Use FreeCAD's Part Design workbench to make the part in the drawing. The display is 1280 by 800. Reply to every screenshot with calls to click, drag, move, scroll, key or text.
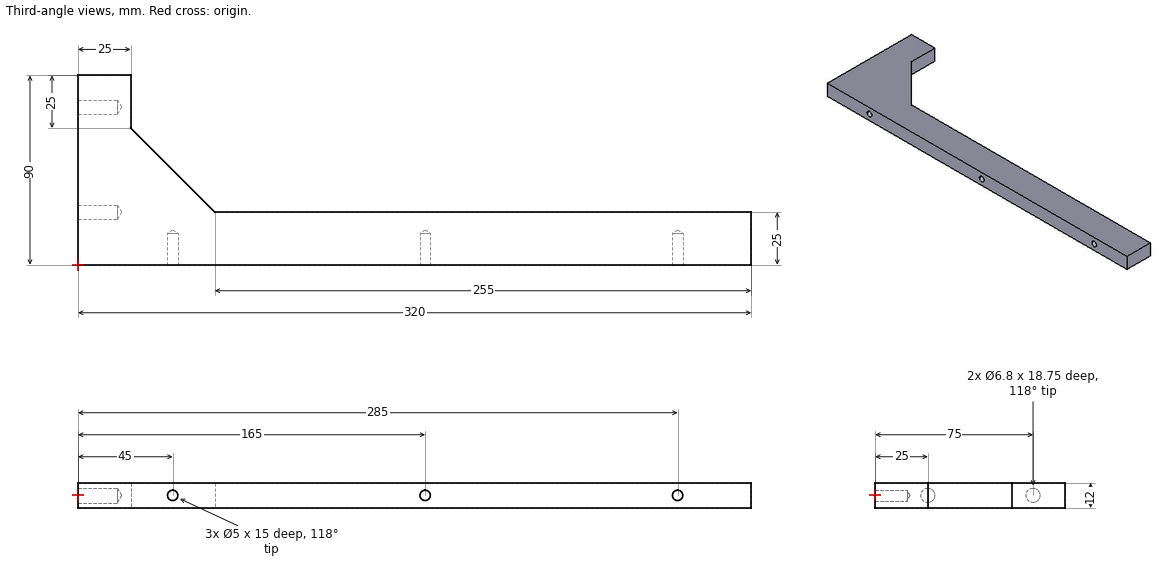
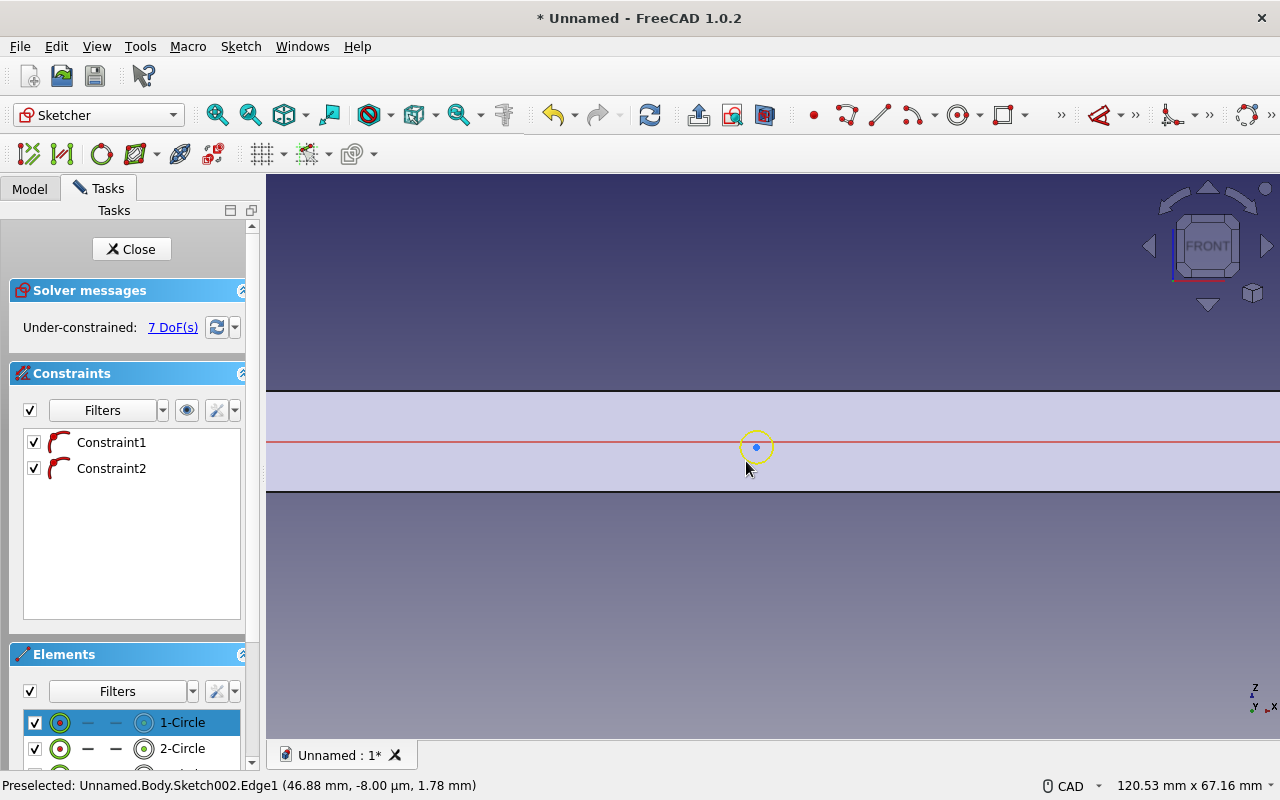
click(745, 459)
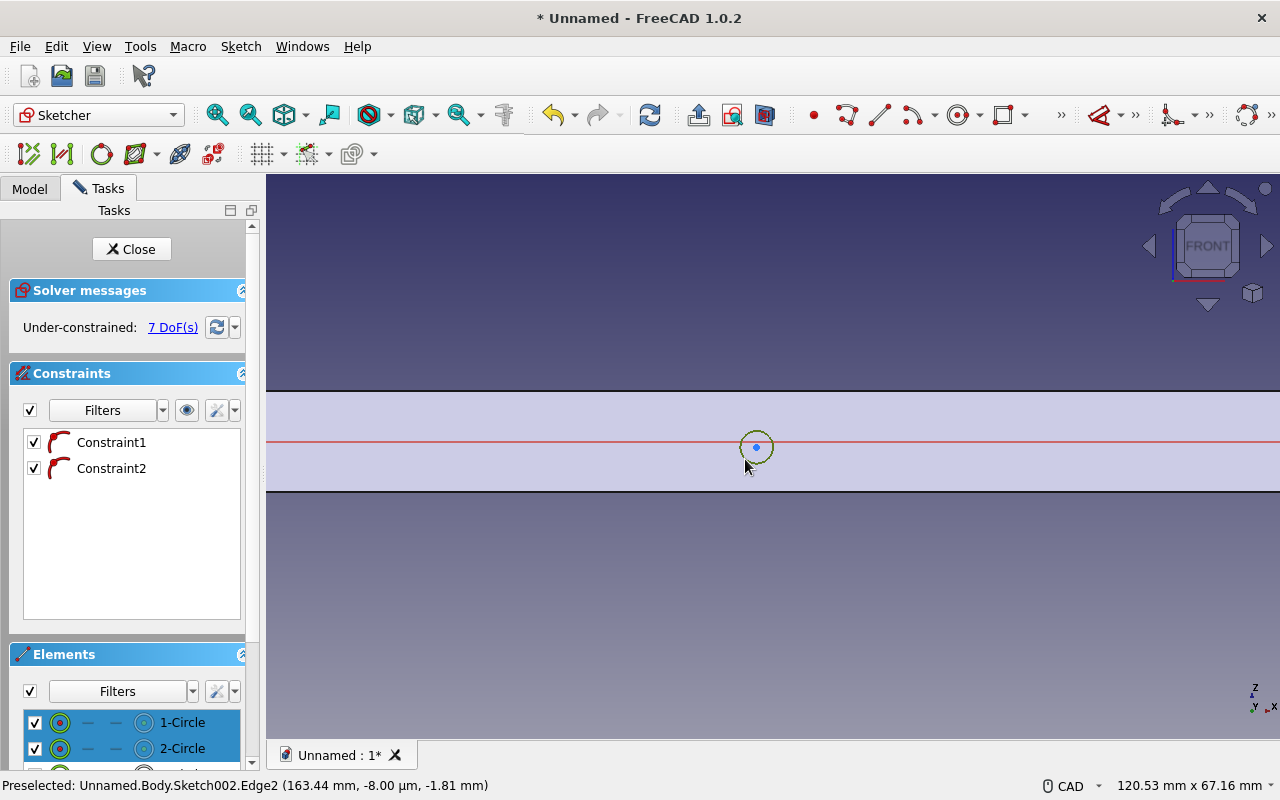
scroll(746, 461, down, 7)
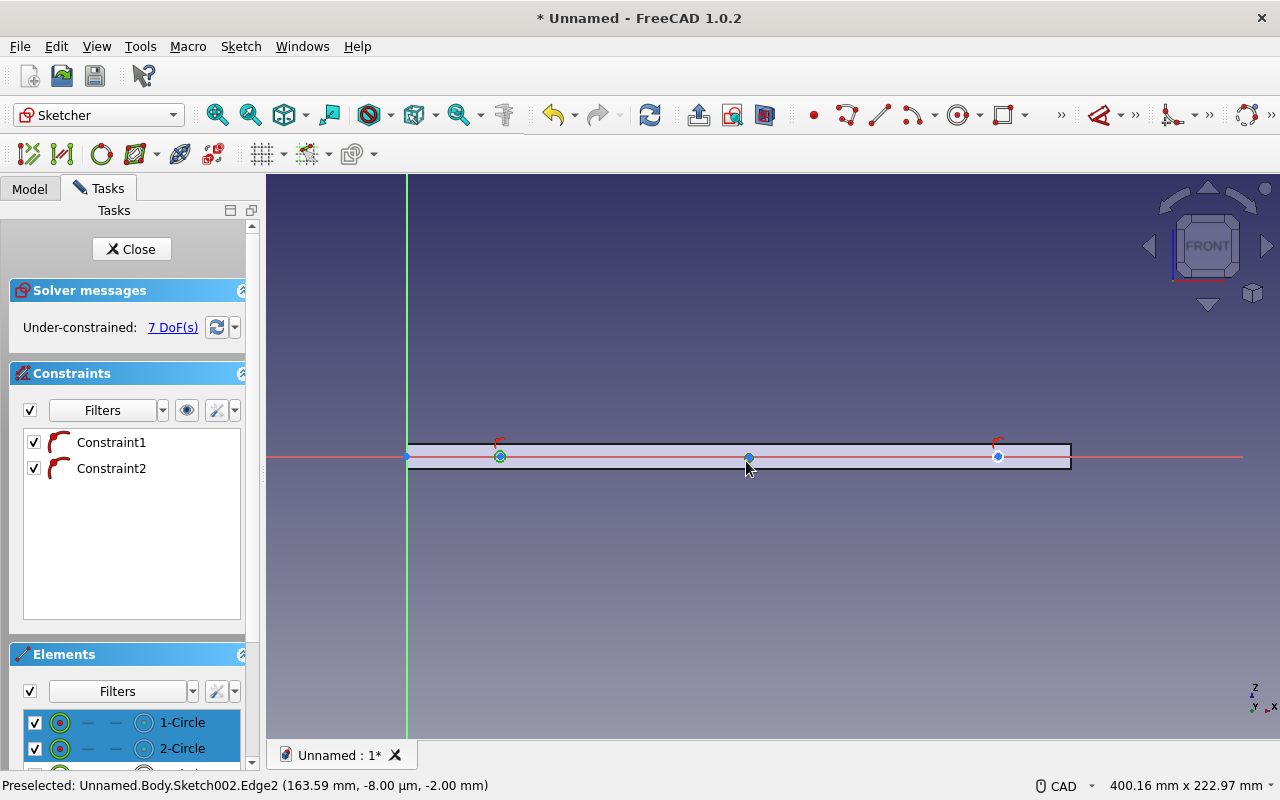
scroll(1002, 453, up, 7)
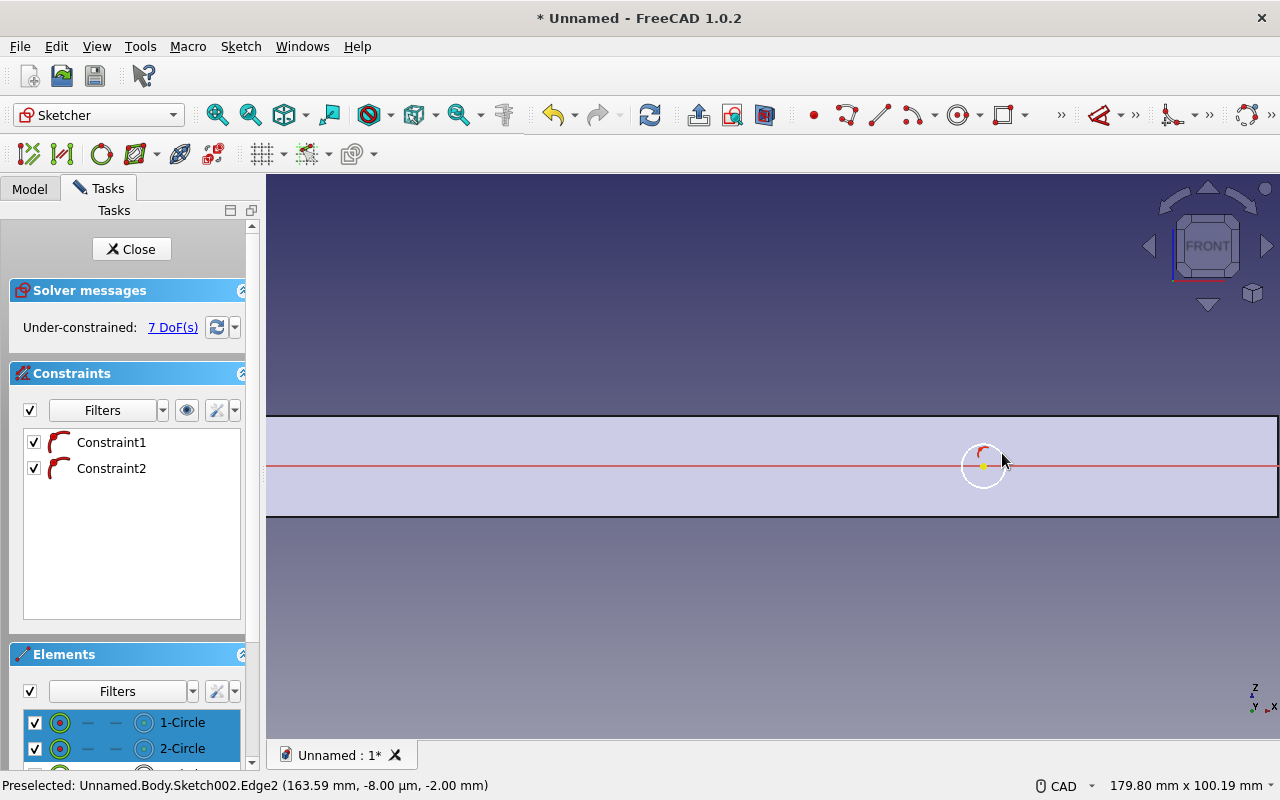
click(999, 451)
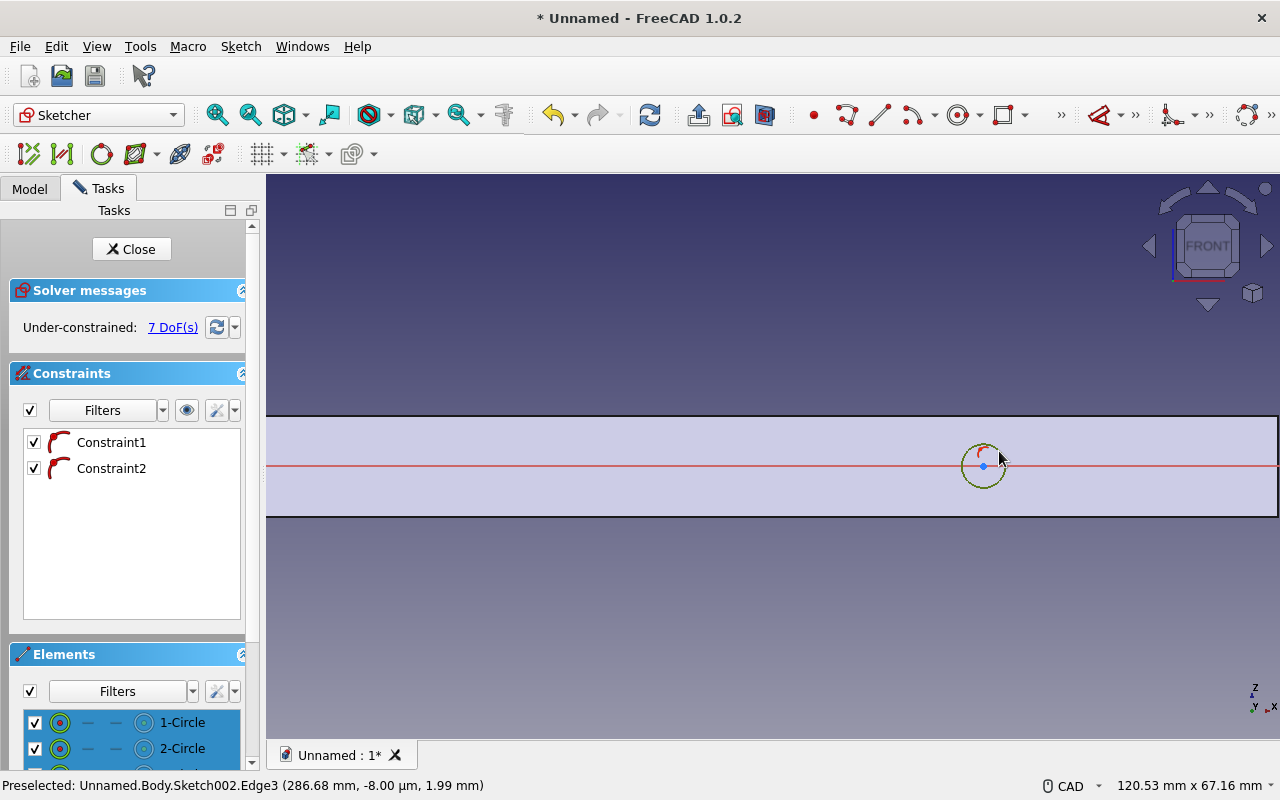
key(e)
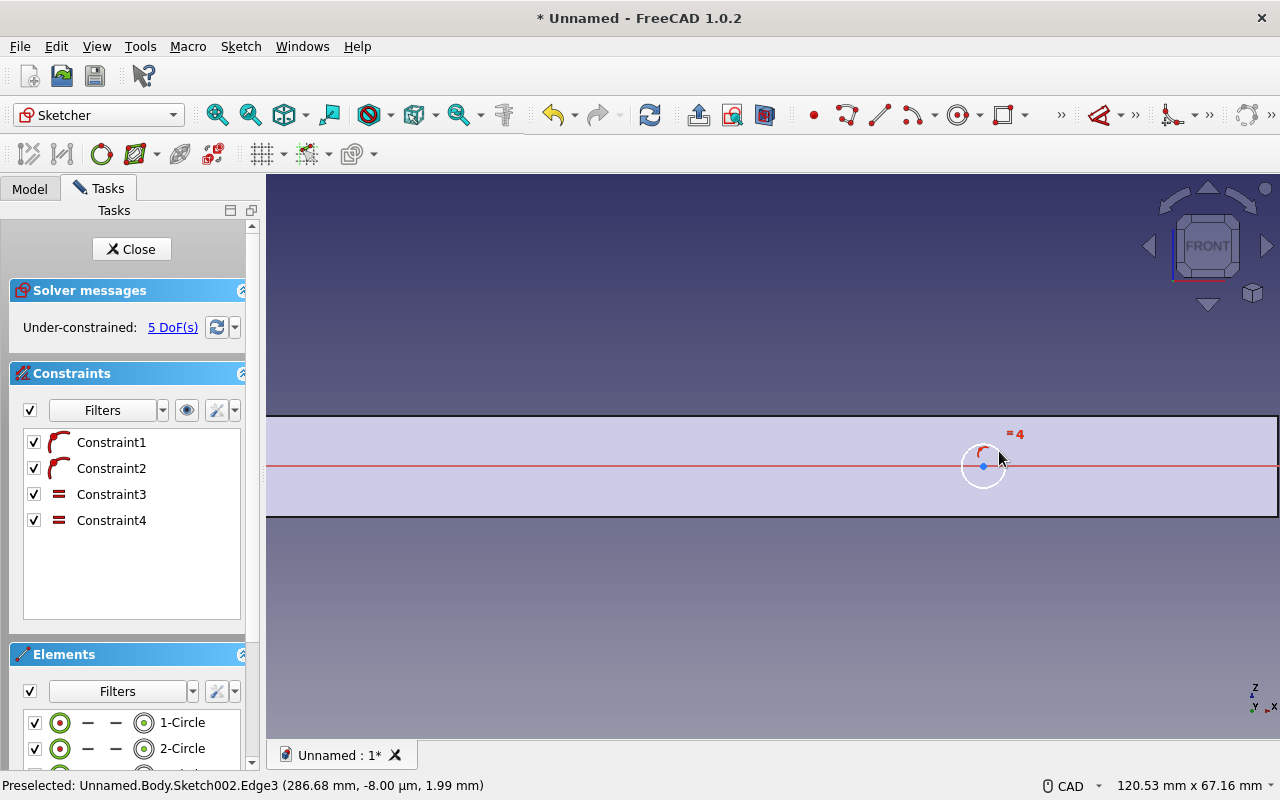
scroll(1002, 453, down, 7)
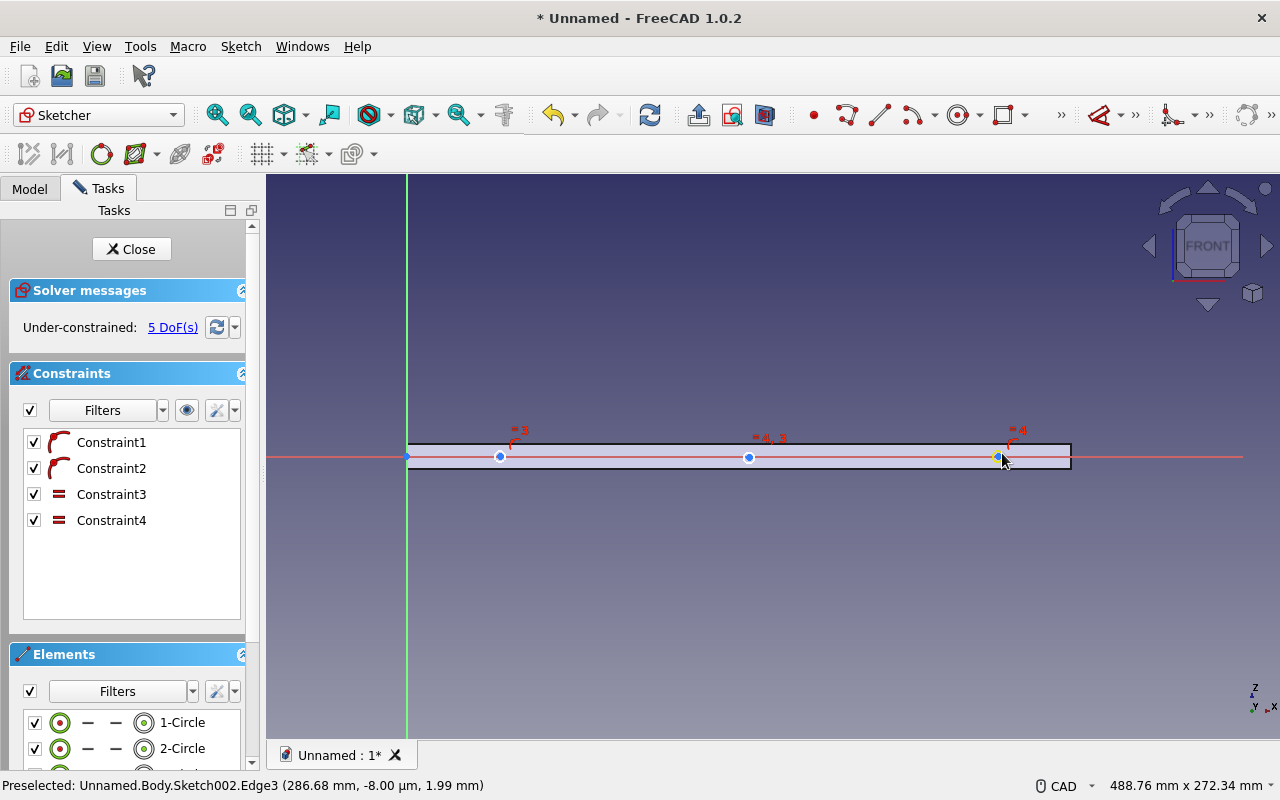
click(749, 458)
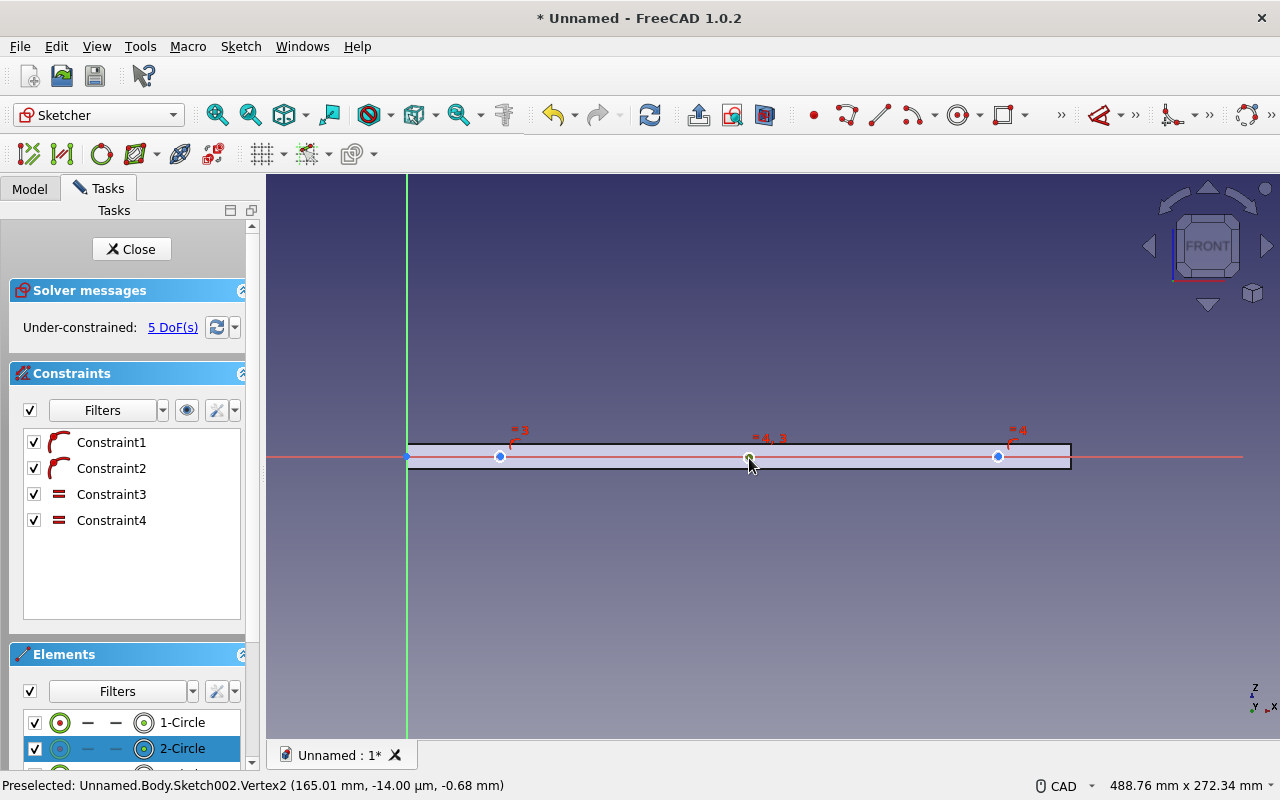
click(353, 457)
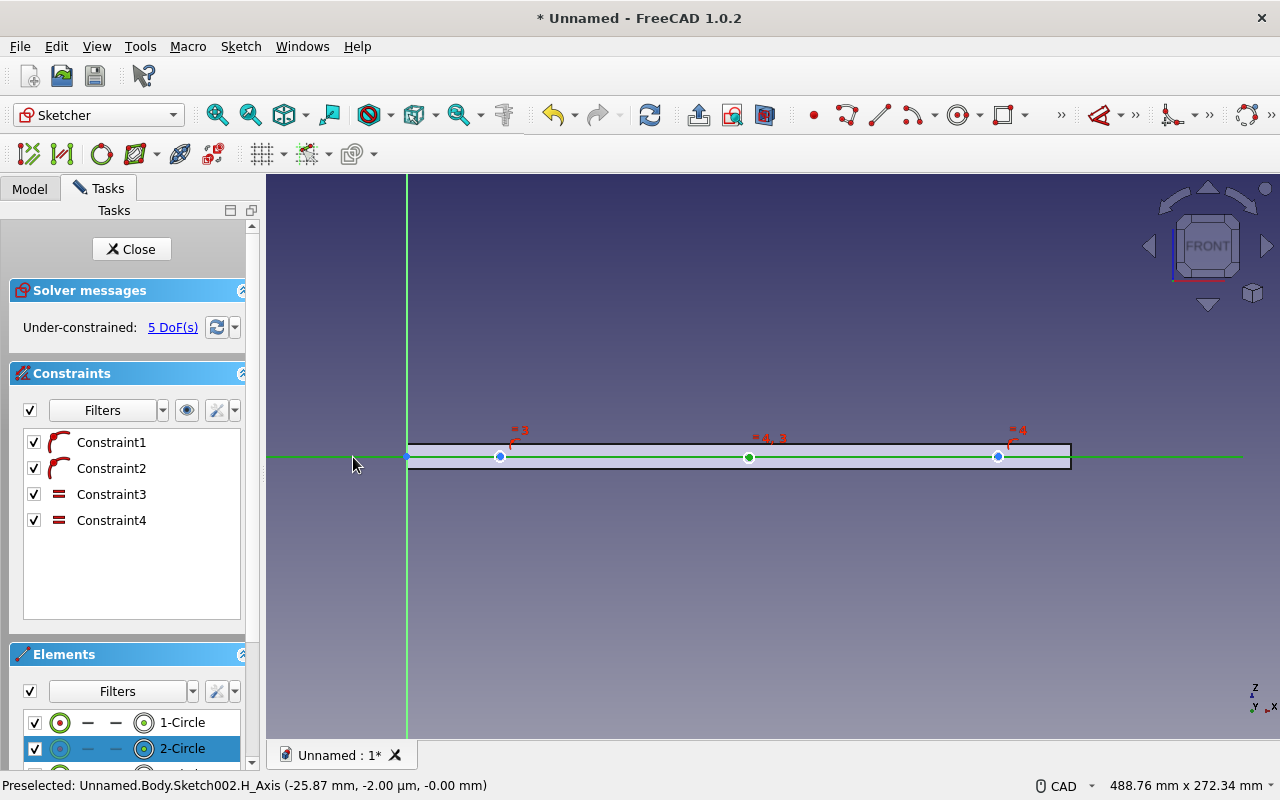
key(c)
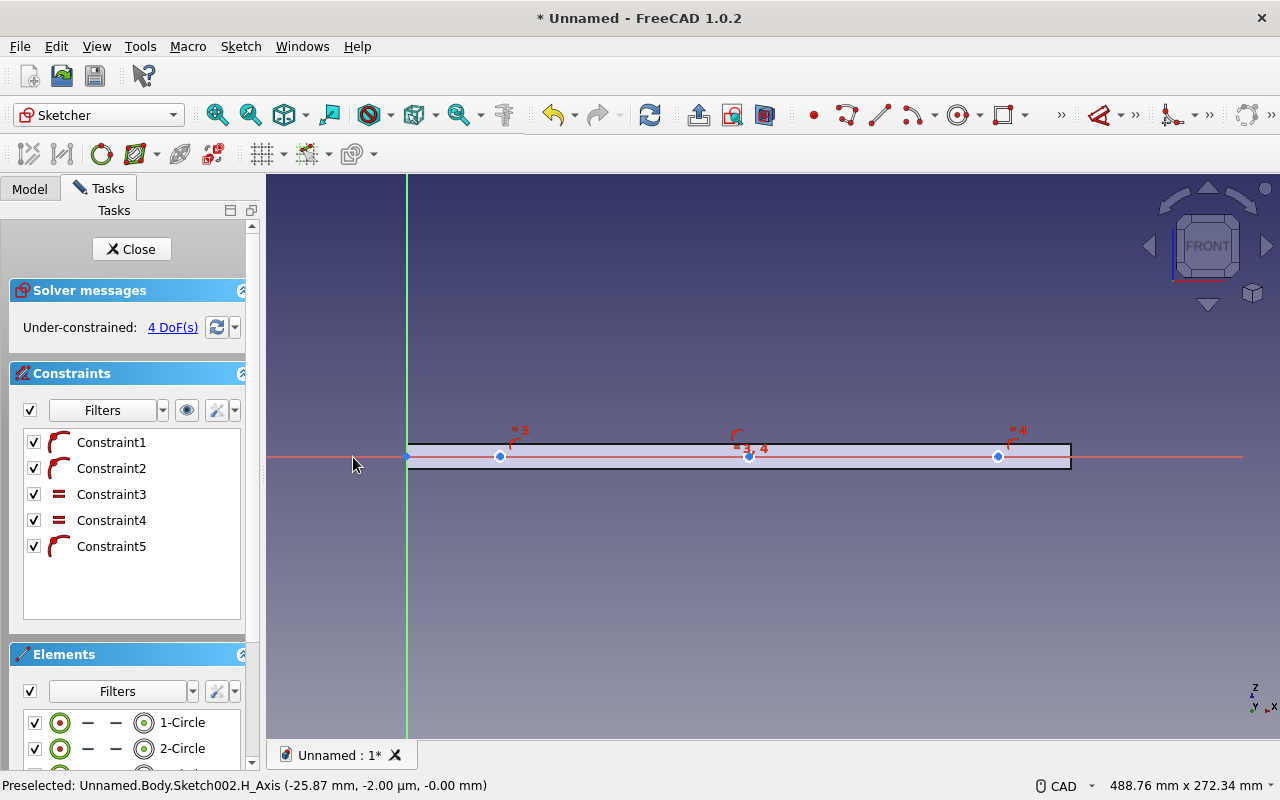
click(1098, 116)